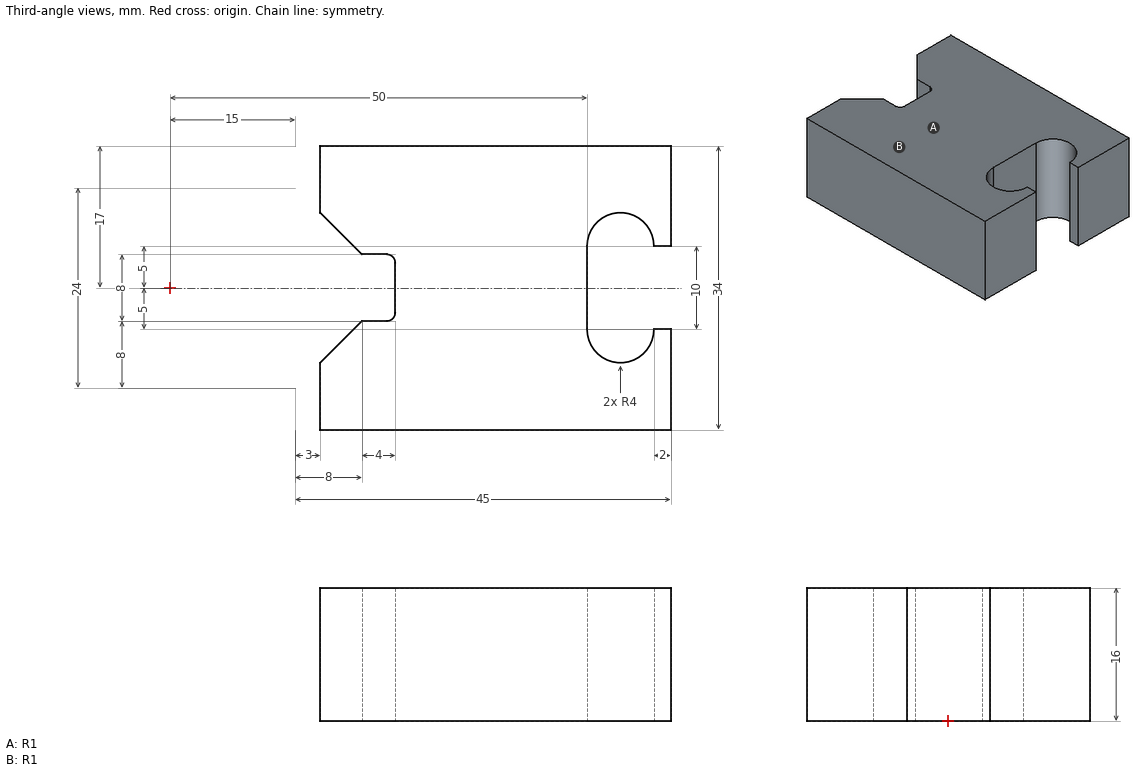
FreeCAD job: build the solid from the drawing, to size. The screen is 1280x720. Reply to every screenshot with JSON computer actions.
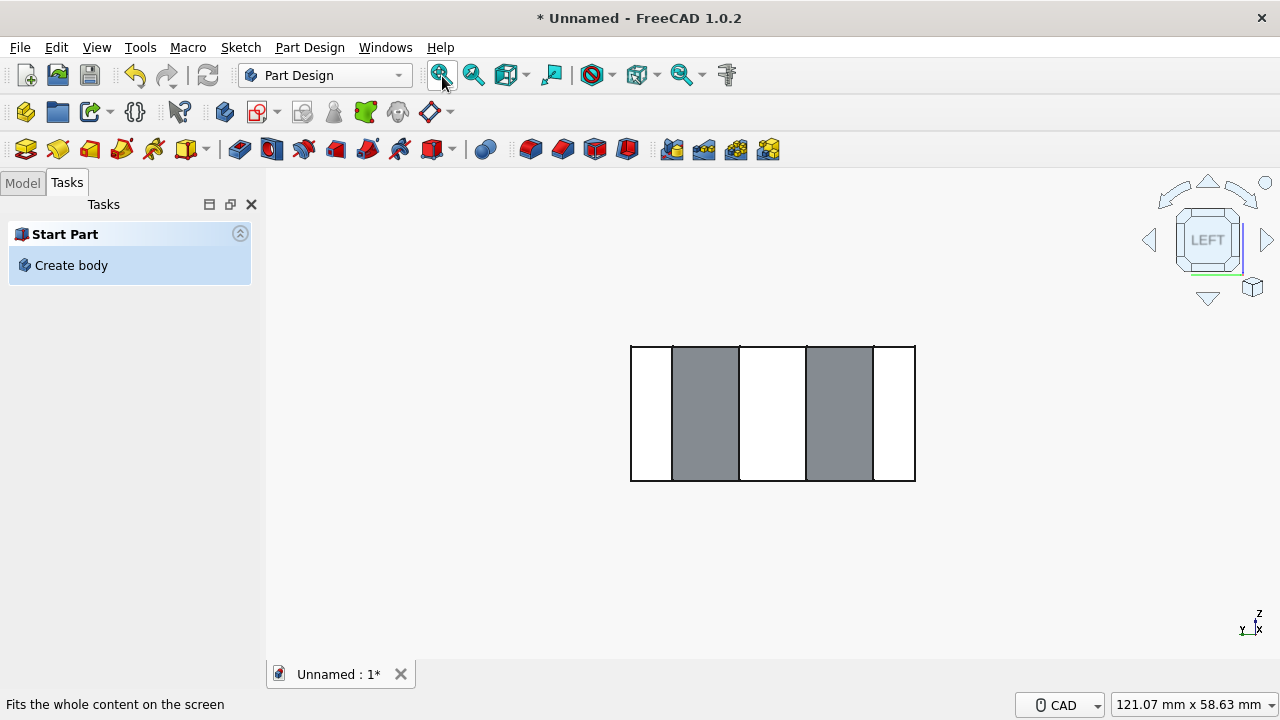
{"action": "key", "text": "v 3"}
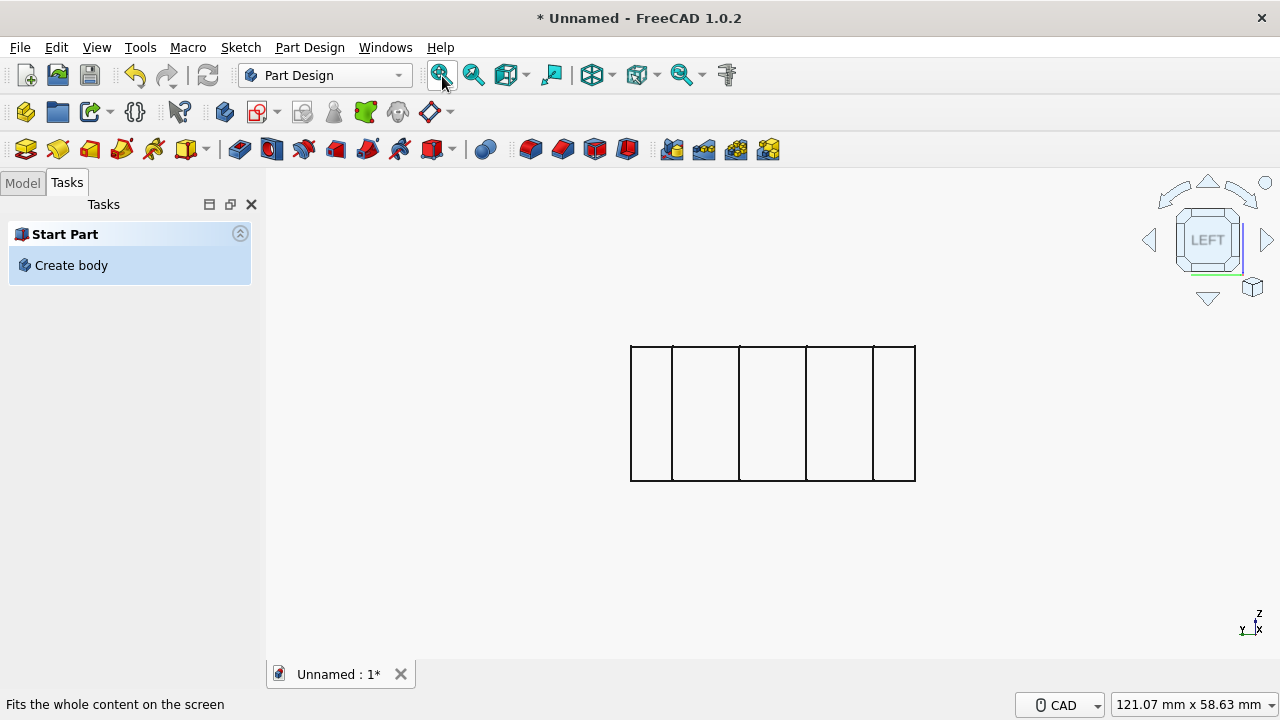
{"action": "key", "text": "0"}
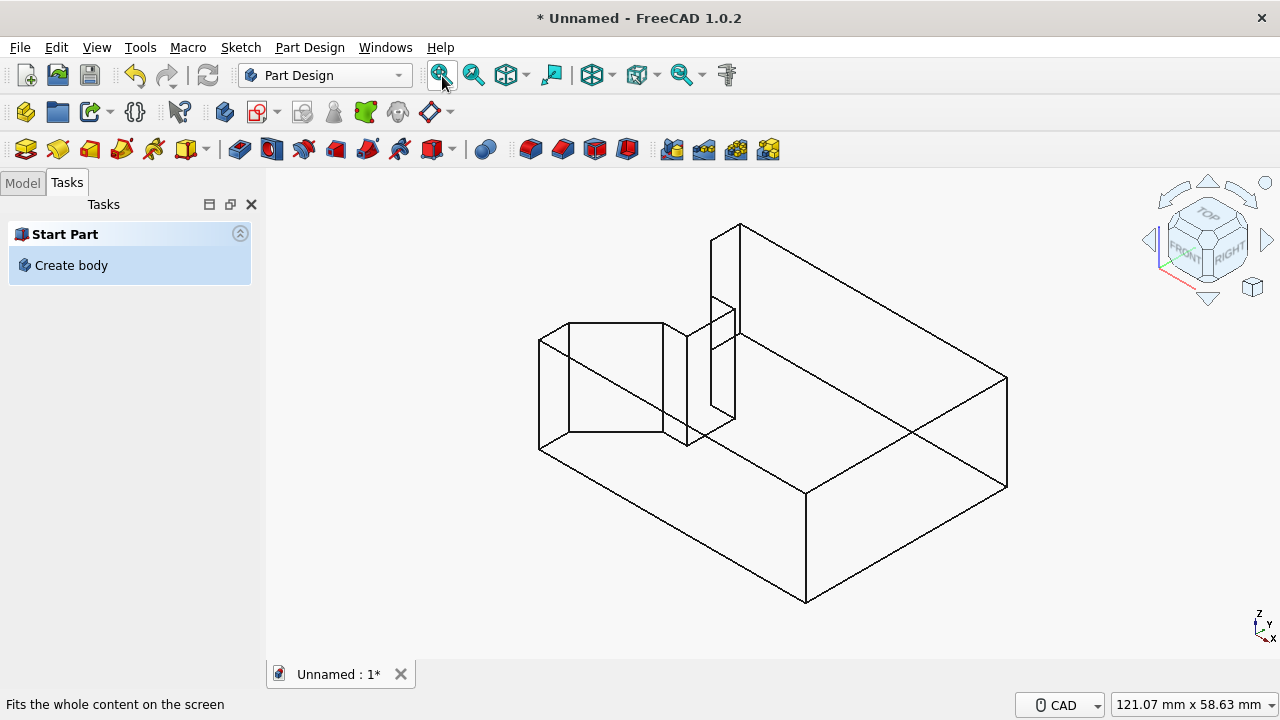
{"action": "left_click", "coordinate": [735, 363]}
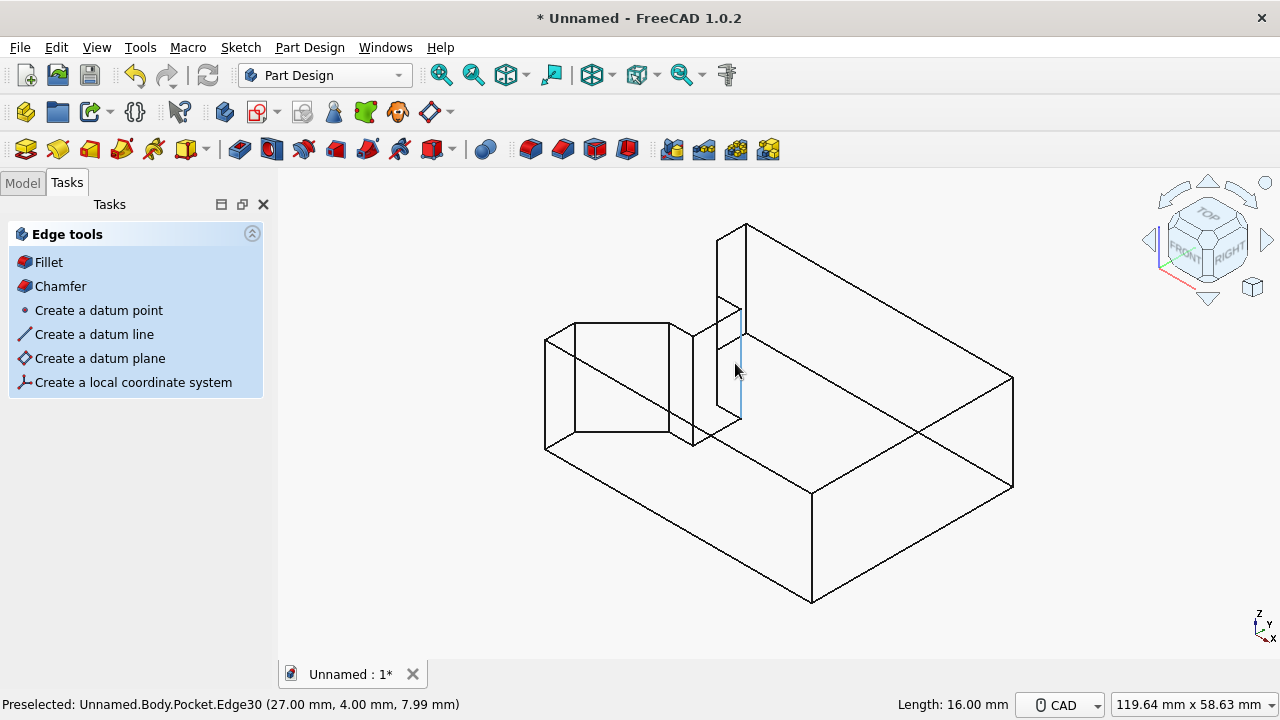
{"action": "key", "text": "v 1"}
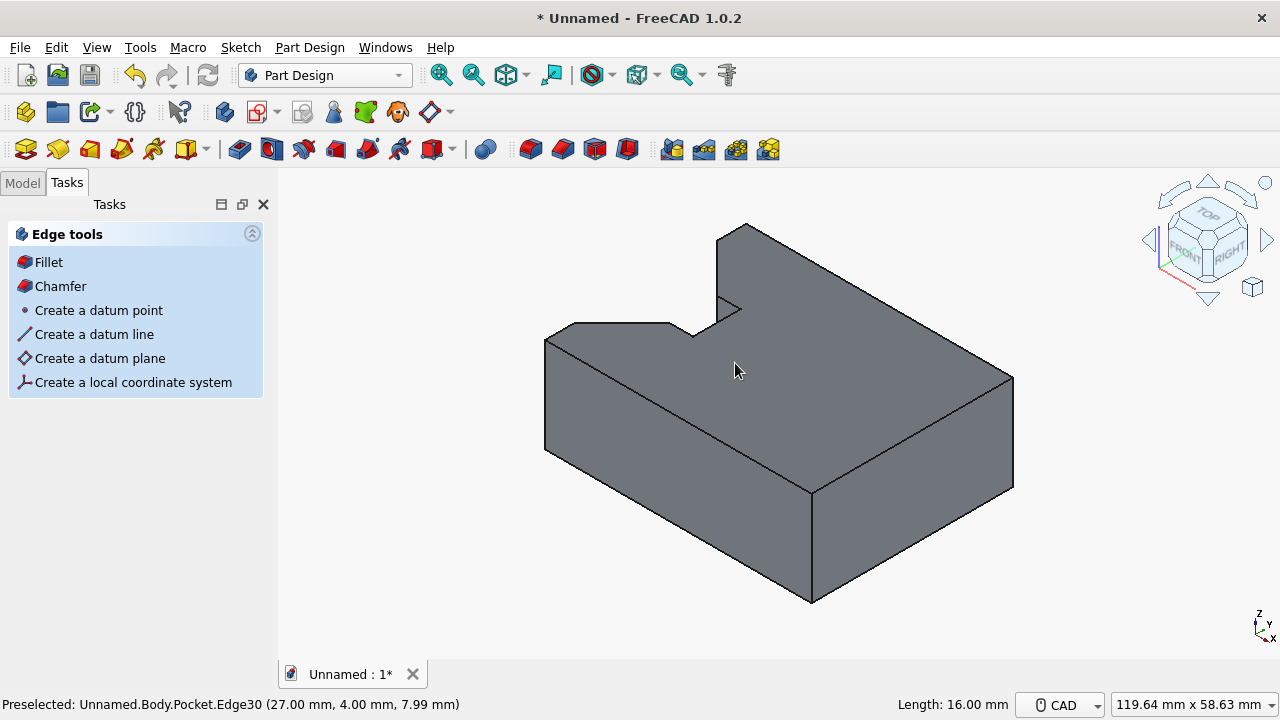
{"action": "left_click", "coordinate": [532, 150]}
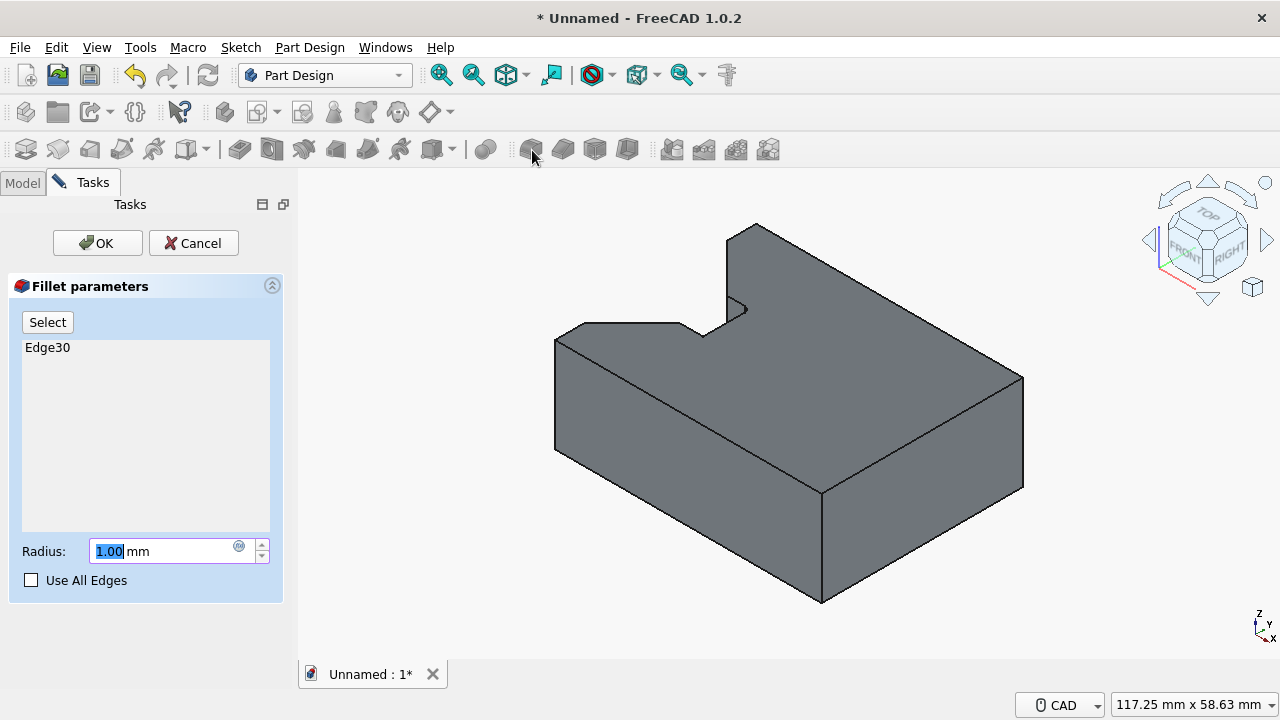
{"action": "type", "text": "1"}
{"action": "key", "text": "Tab"}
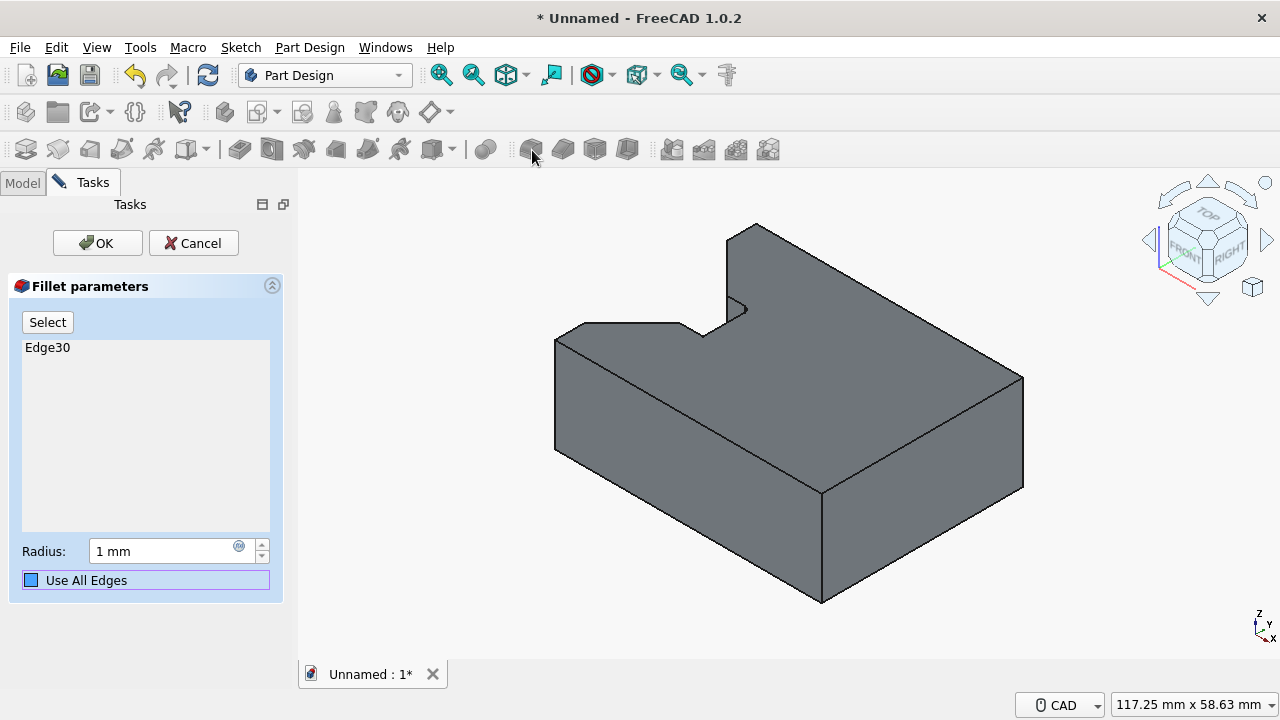
{"action": "left_click", "coordinate": [98, 243]}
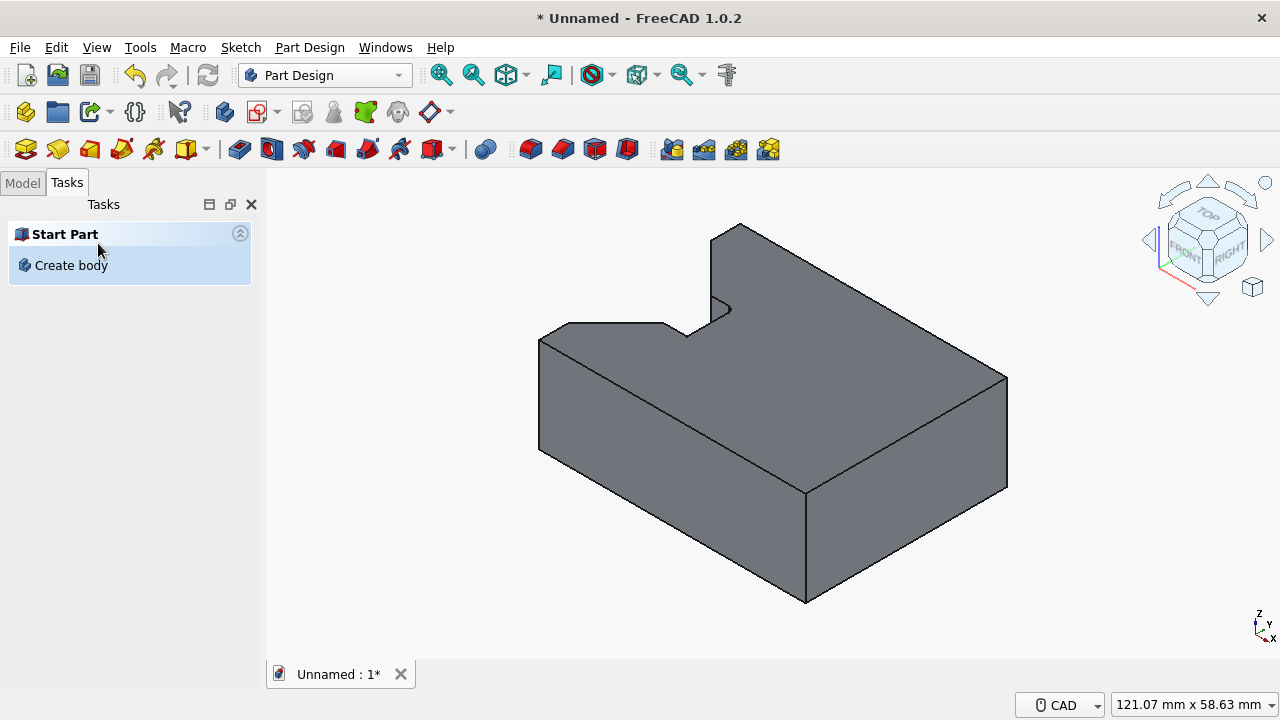
{"action": "key", "text": "2"}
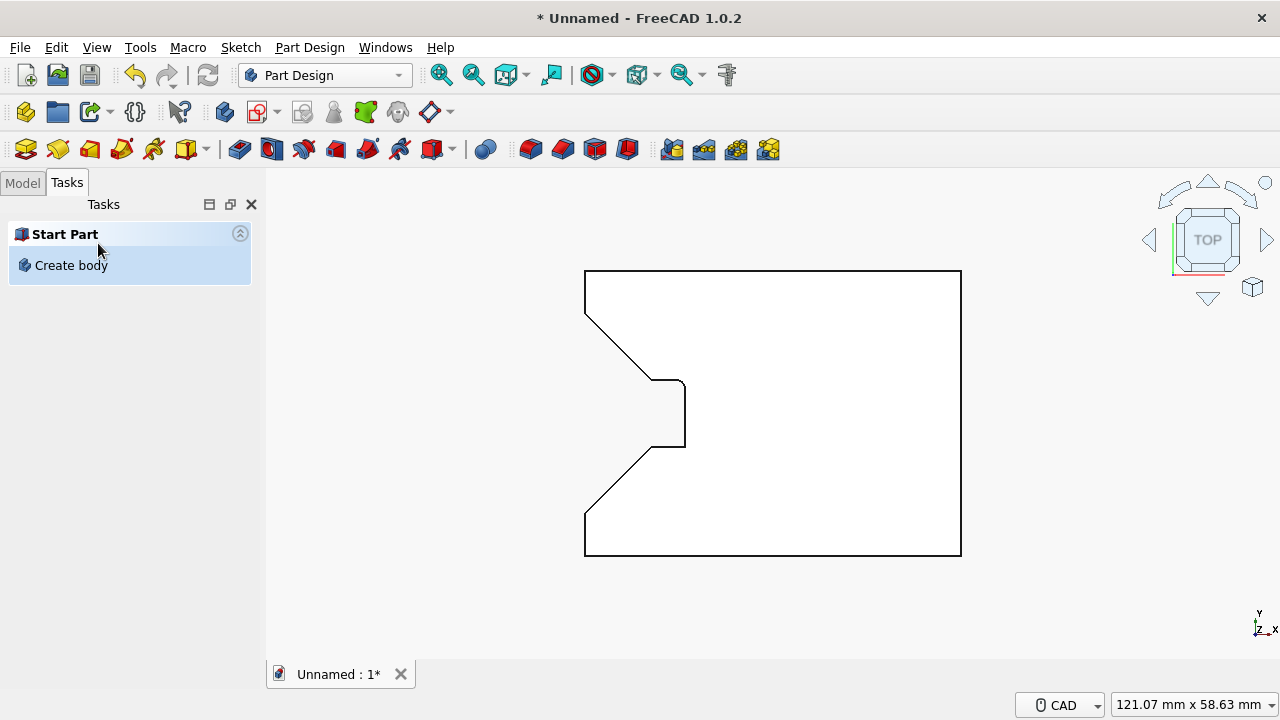
{"action": "key", "text": "0"}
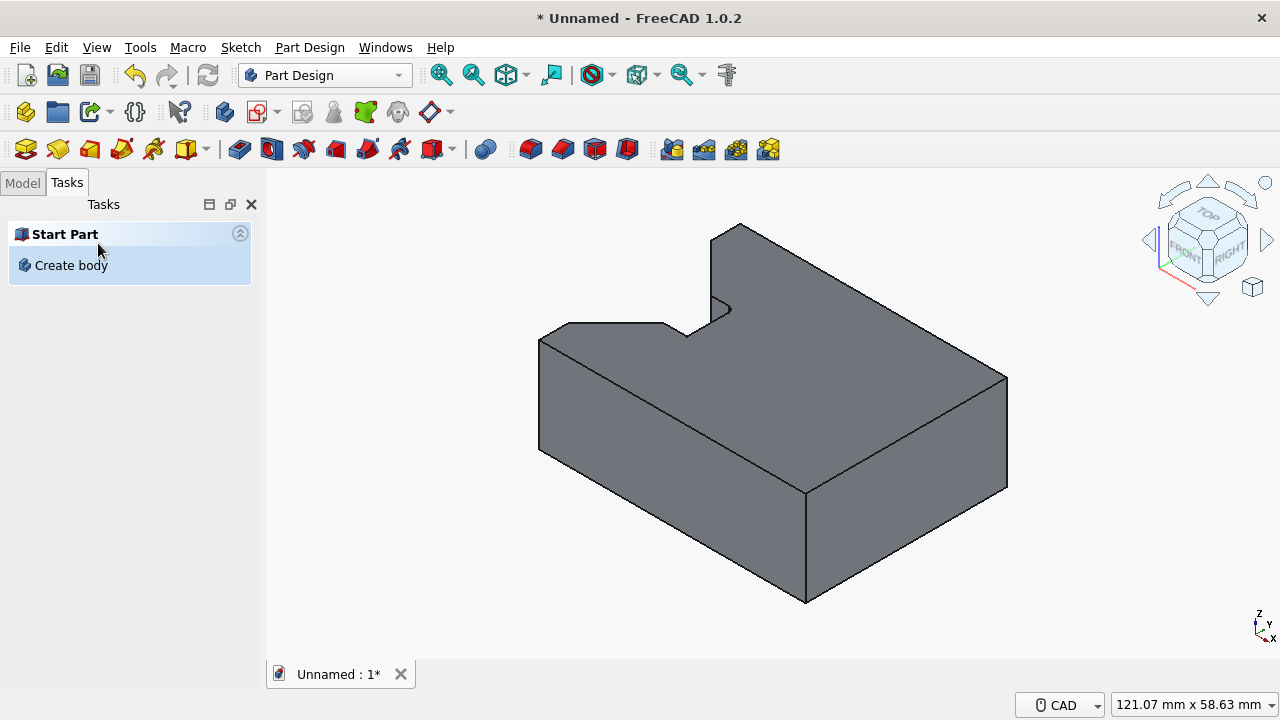
{"action": "key", "text": "1"}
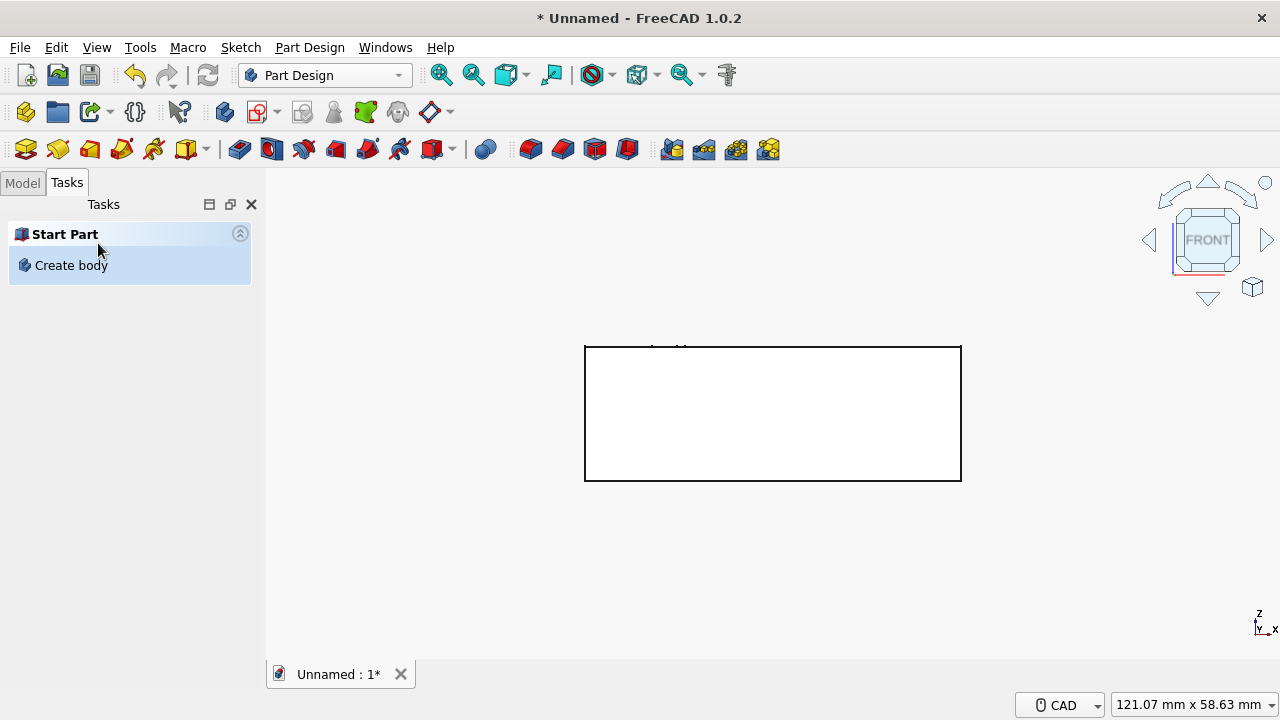
{"action": "left_click", "coordinate": [442, 76]}